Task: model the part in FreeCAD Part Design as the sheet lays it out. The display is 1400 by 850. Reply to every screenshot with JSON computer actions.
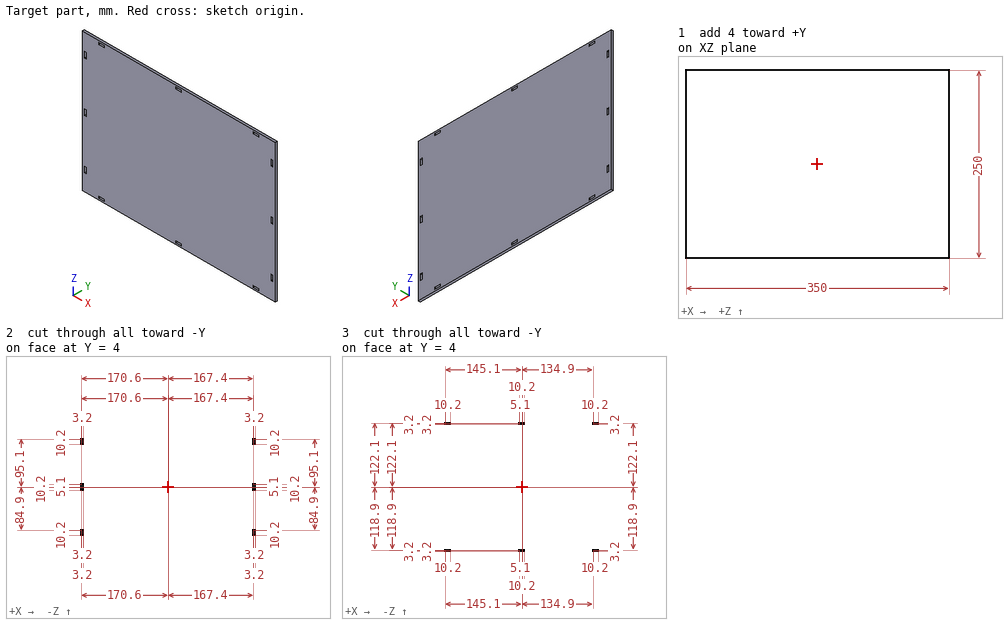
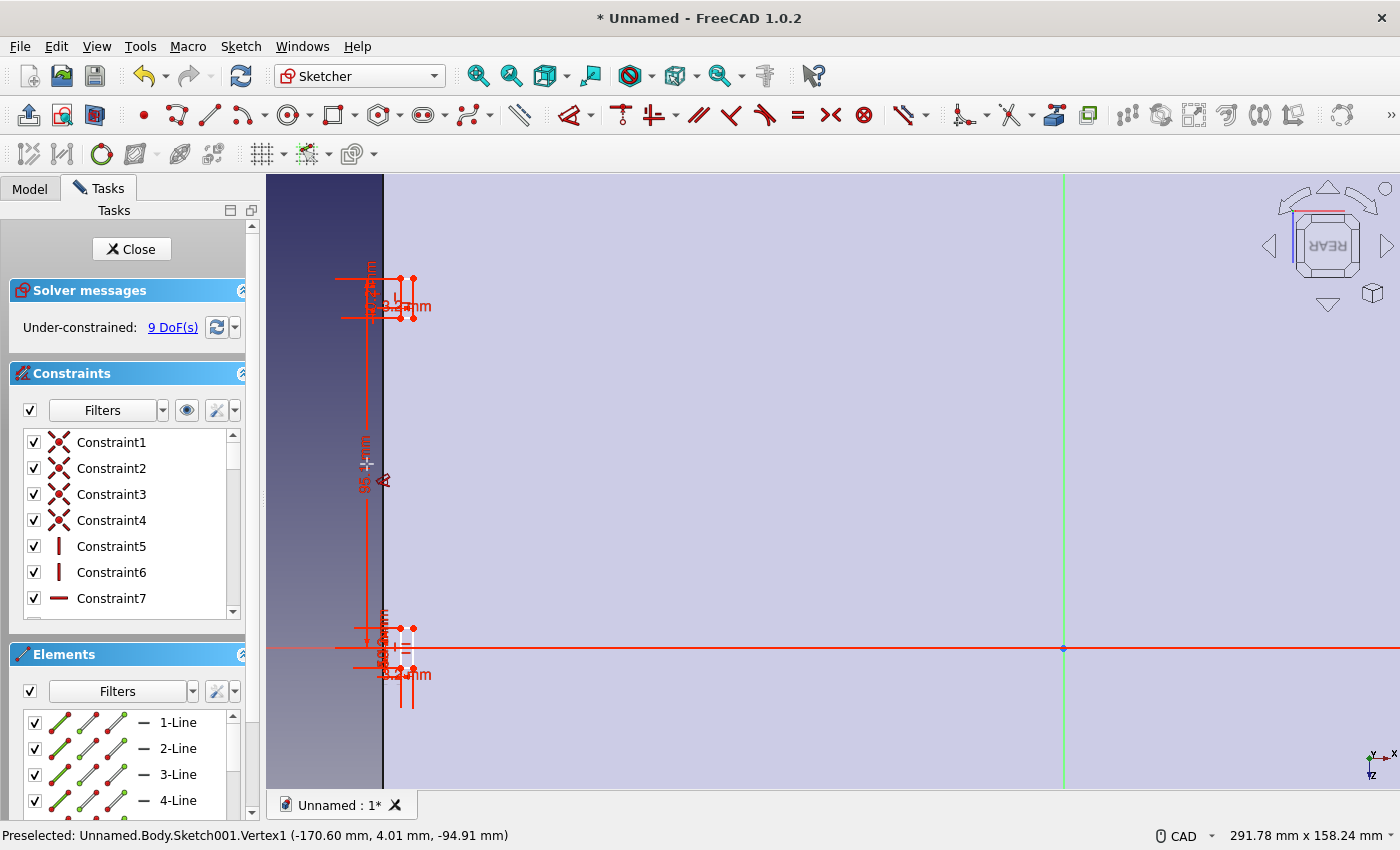
{"action": "scroll", "coordinate": [401, 279], "scroll_direction": "down", "scroll_amount": 3}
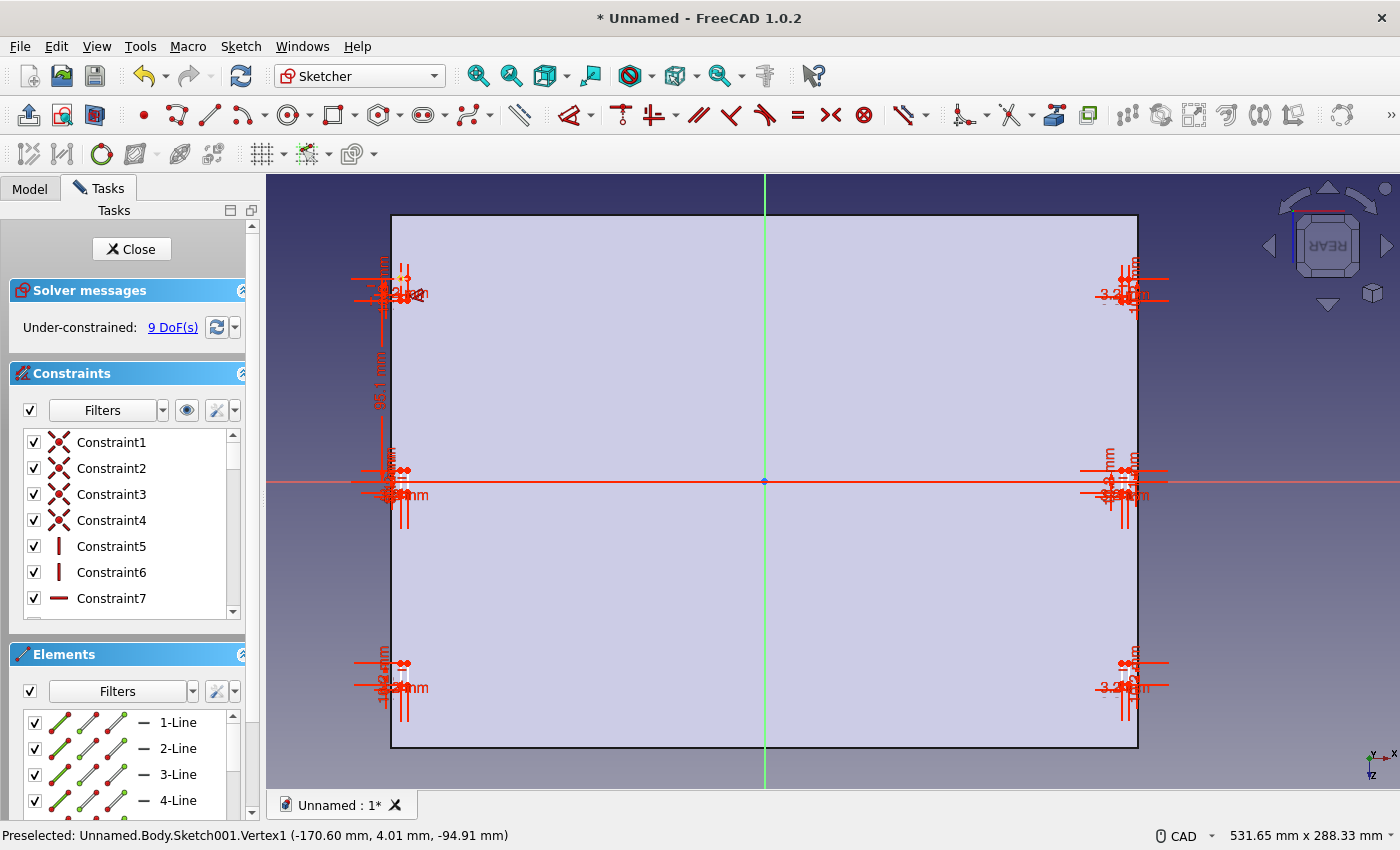
{"action": "scroll", "coordinate": [401, 663], "scroll_direction": "up", "scroll_amount": 3}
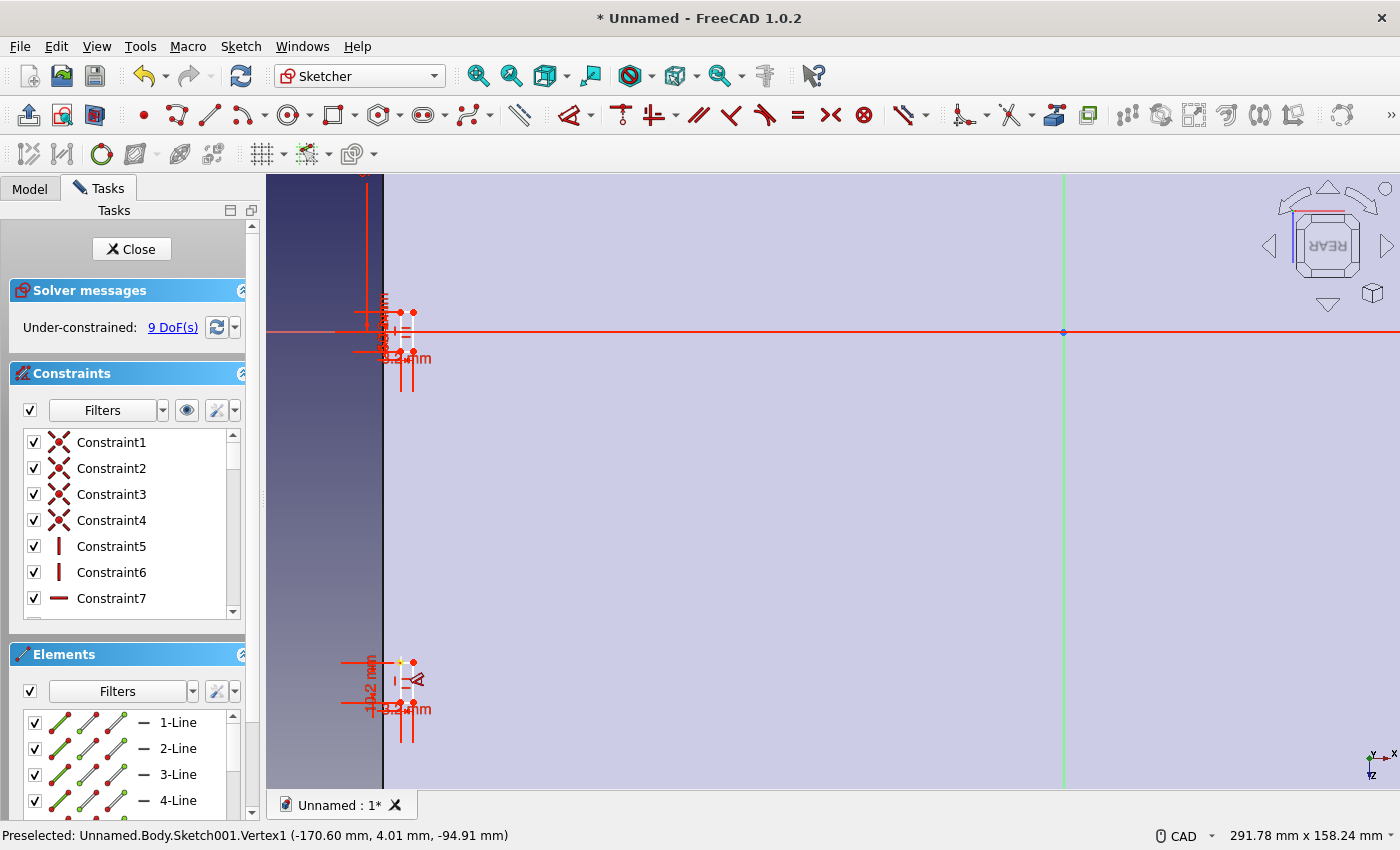
{"action": "left_click", "coordinate": [401, 663]}
{"action": "left_click", "coordinate": [367, 498]}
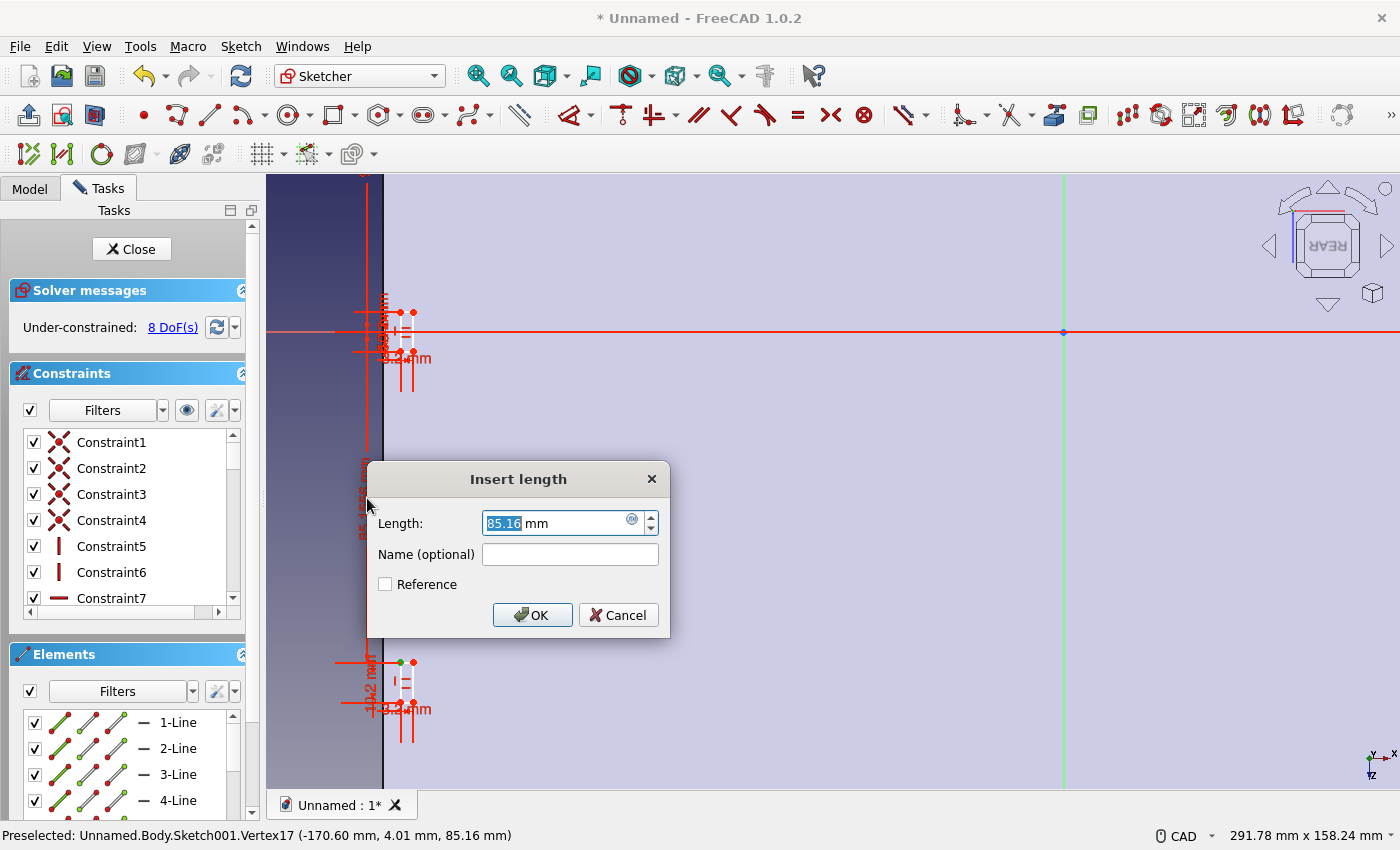
{"action": "type", "text": "84.9"}
{"action": "key", "text": "Return"}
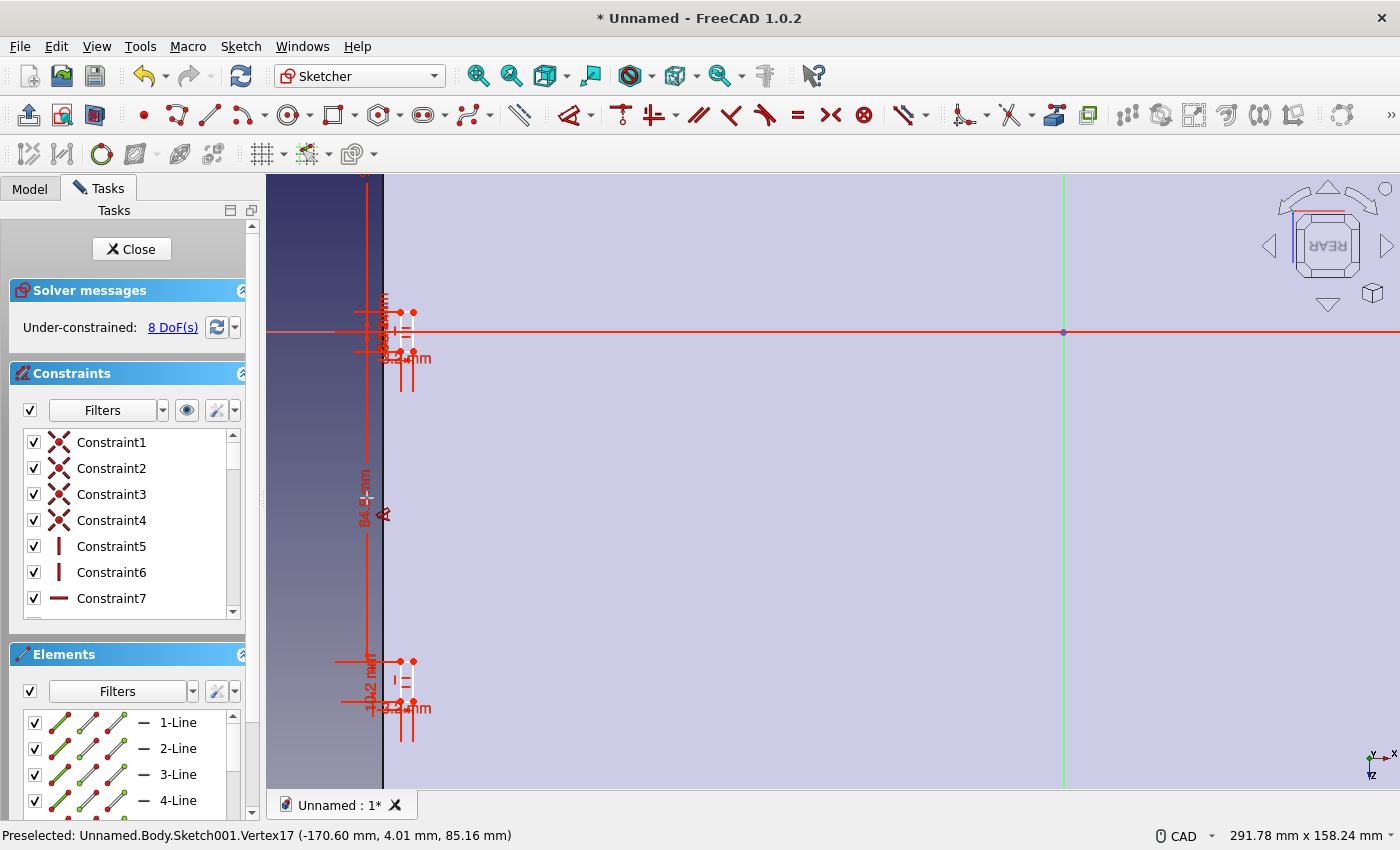
{"action": "scroll", "coordinate": [401, 663], "scroll_direction": "down", "scroll_amount": 3}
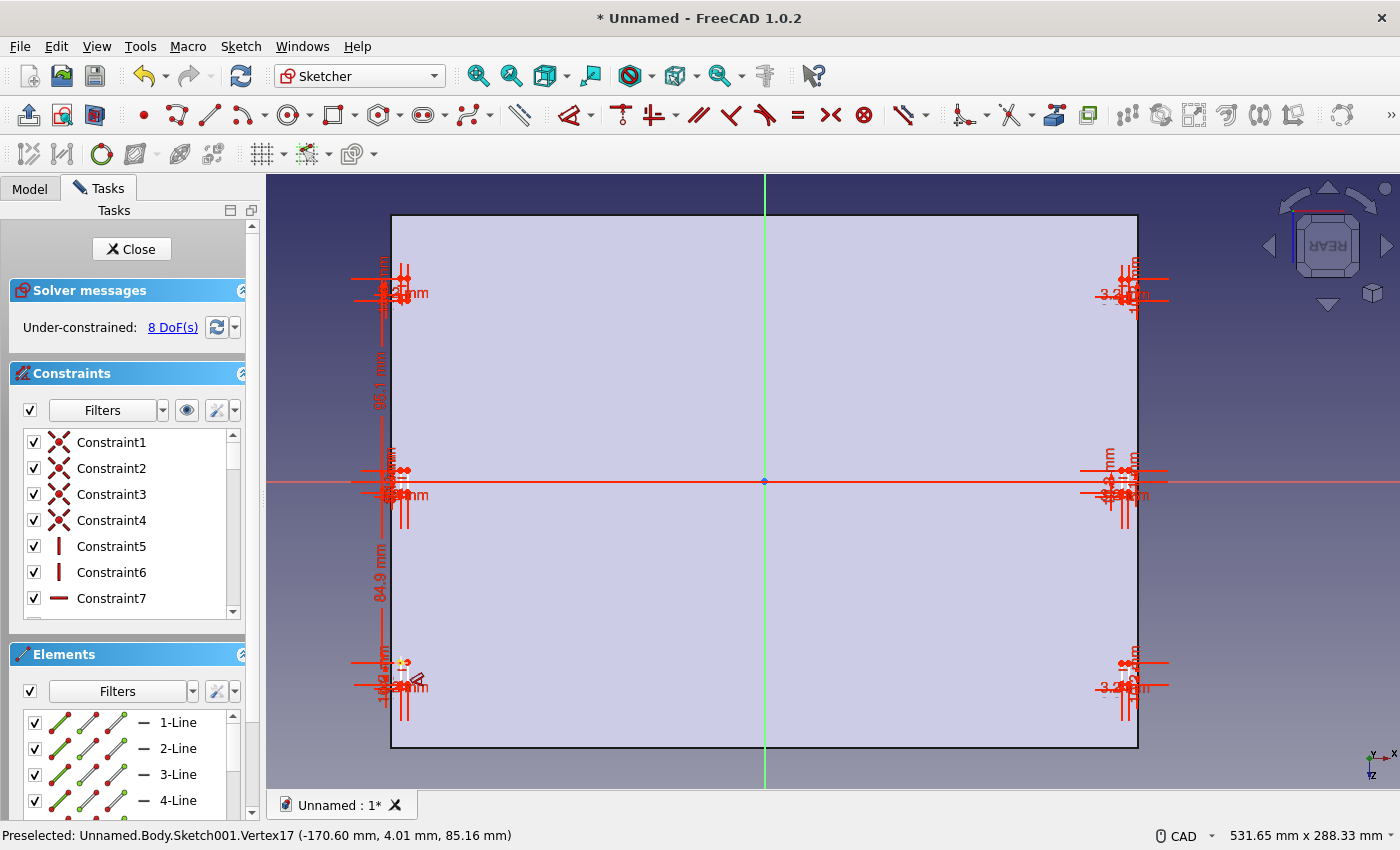
{"action": "scroll", "coordinate": [1122, 663], "scroll_direction": "up", "scroll_amount": 3}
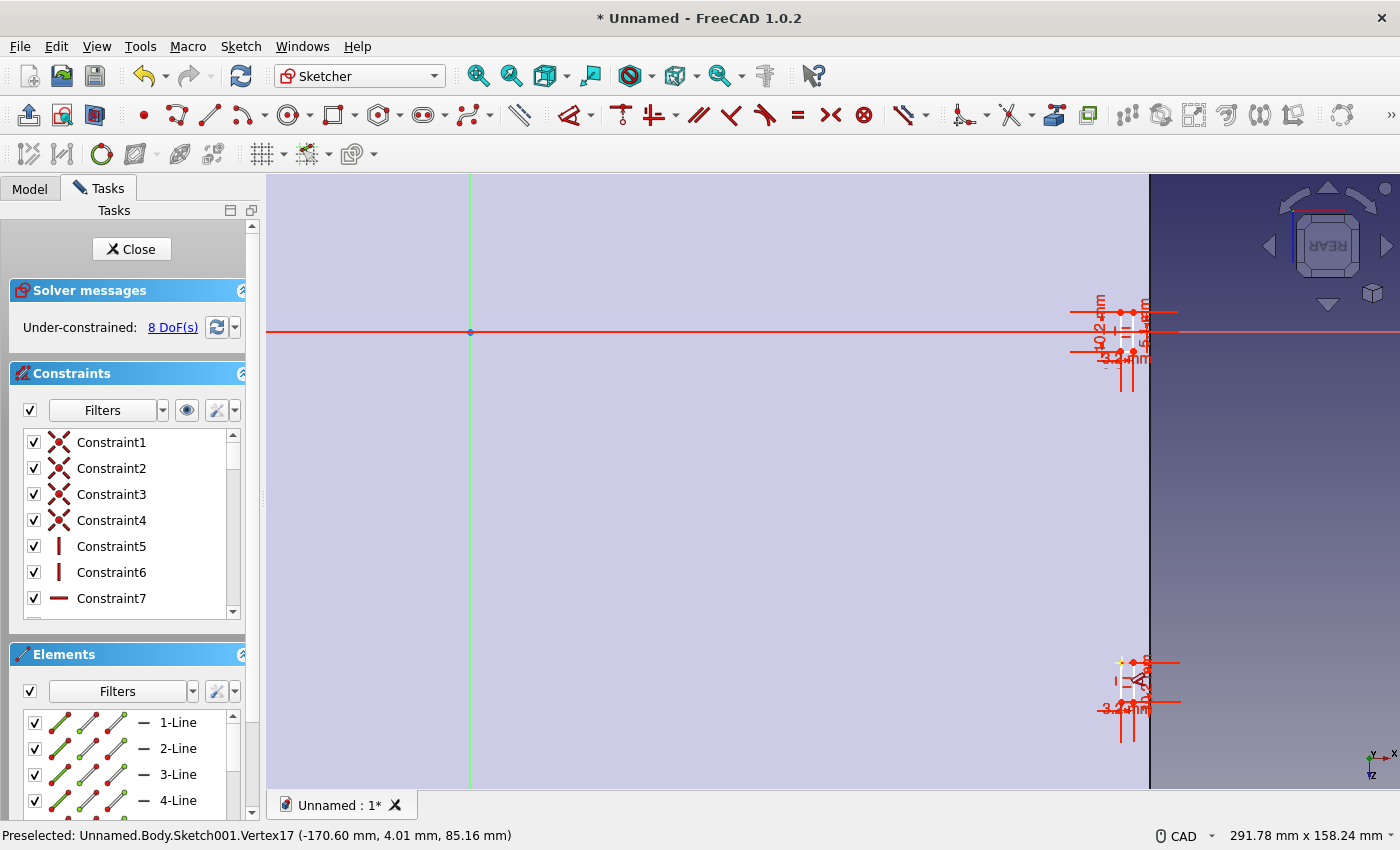
{"action": "left_click", "coordinate": [1121, 663]}
{"action": "left_click", "coordinate": [1155, 497]}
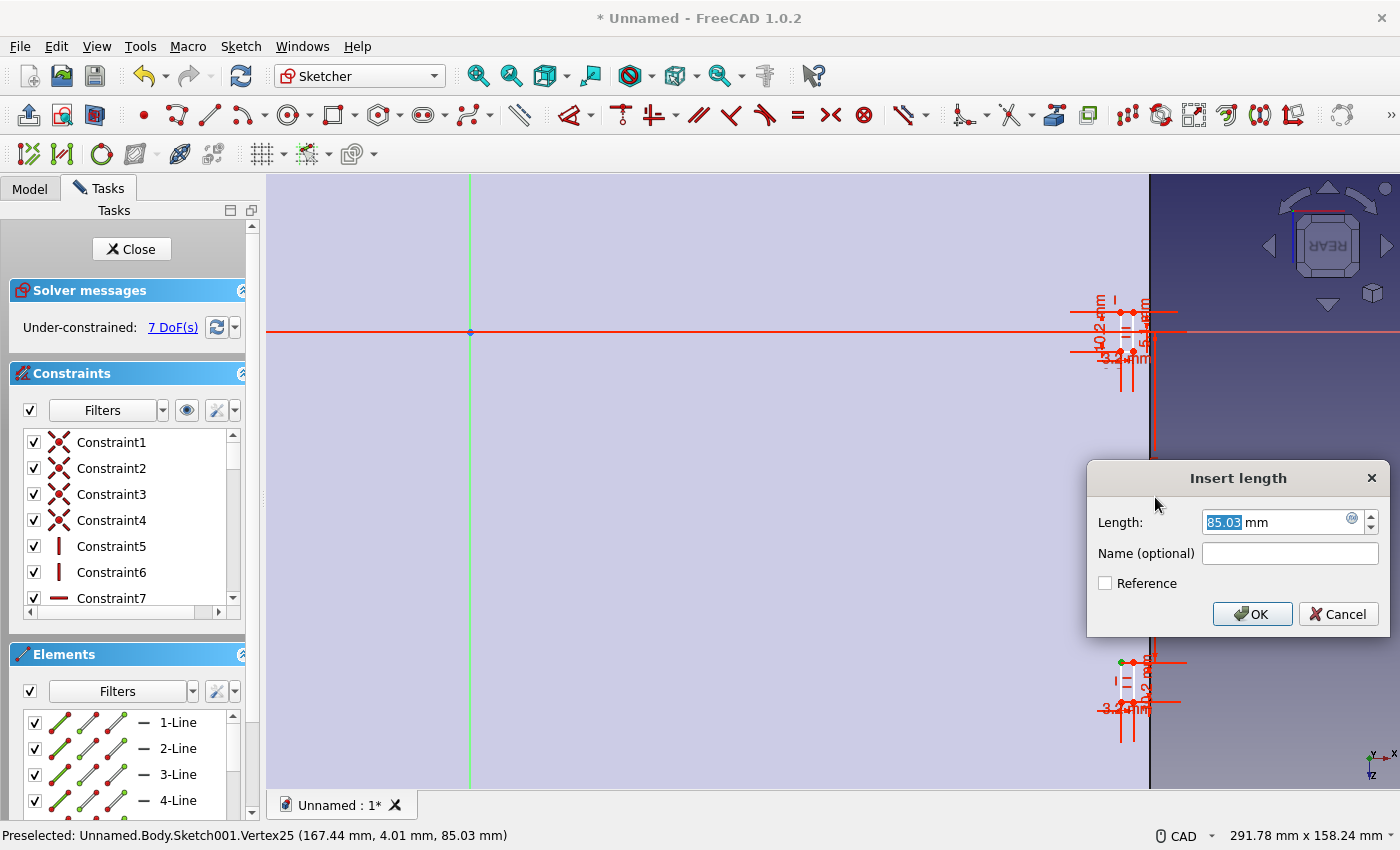
{"action": "type", "text": "84.9"}
{"action": "key", "text": "Return"}